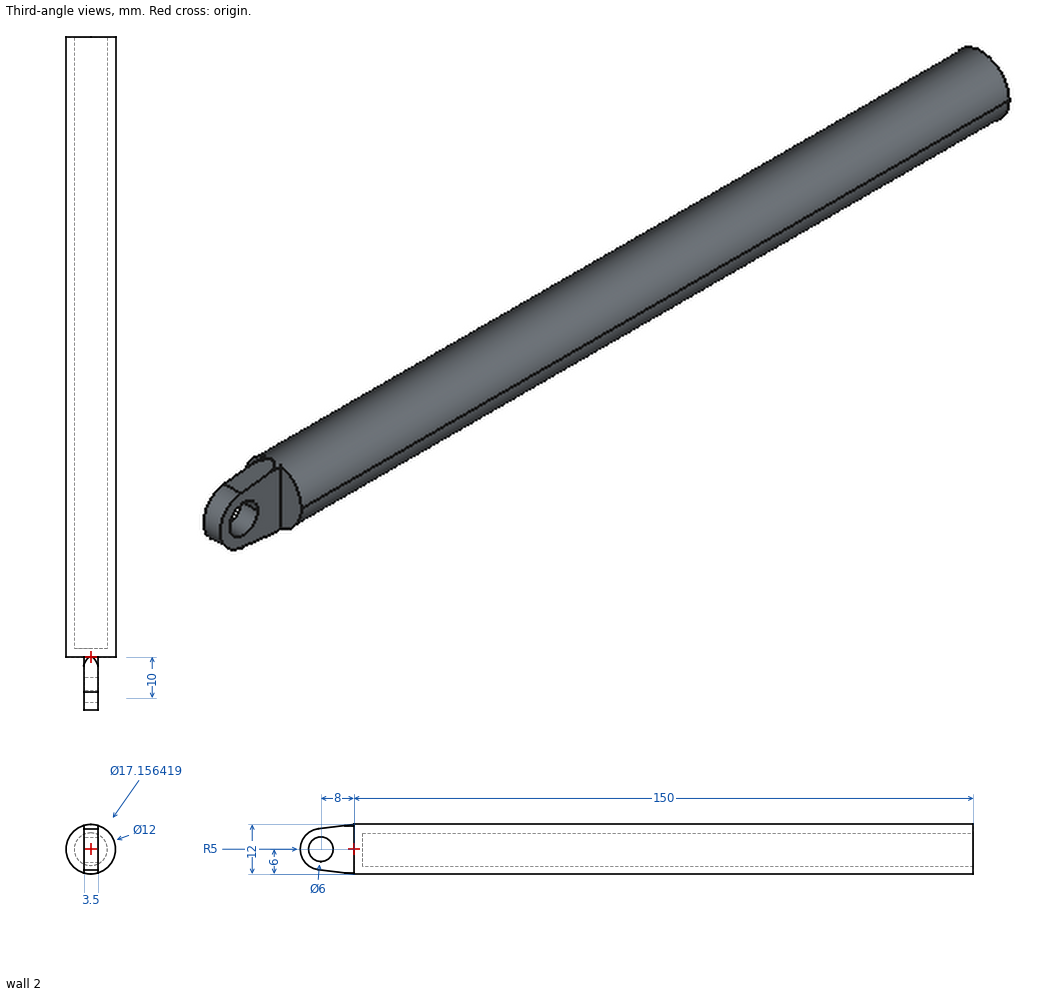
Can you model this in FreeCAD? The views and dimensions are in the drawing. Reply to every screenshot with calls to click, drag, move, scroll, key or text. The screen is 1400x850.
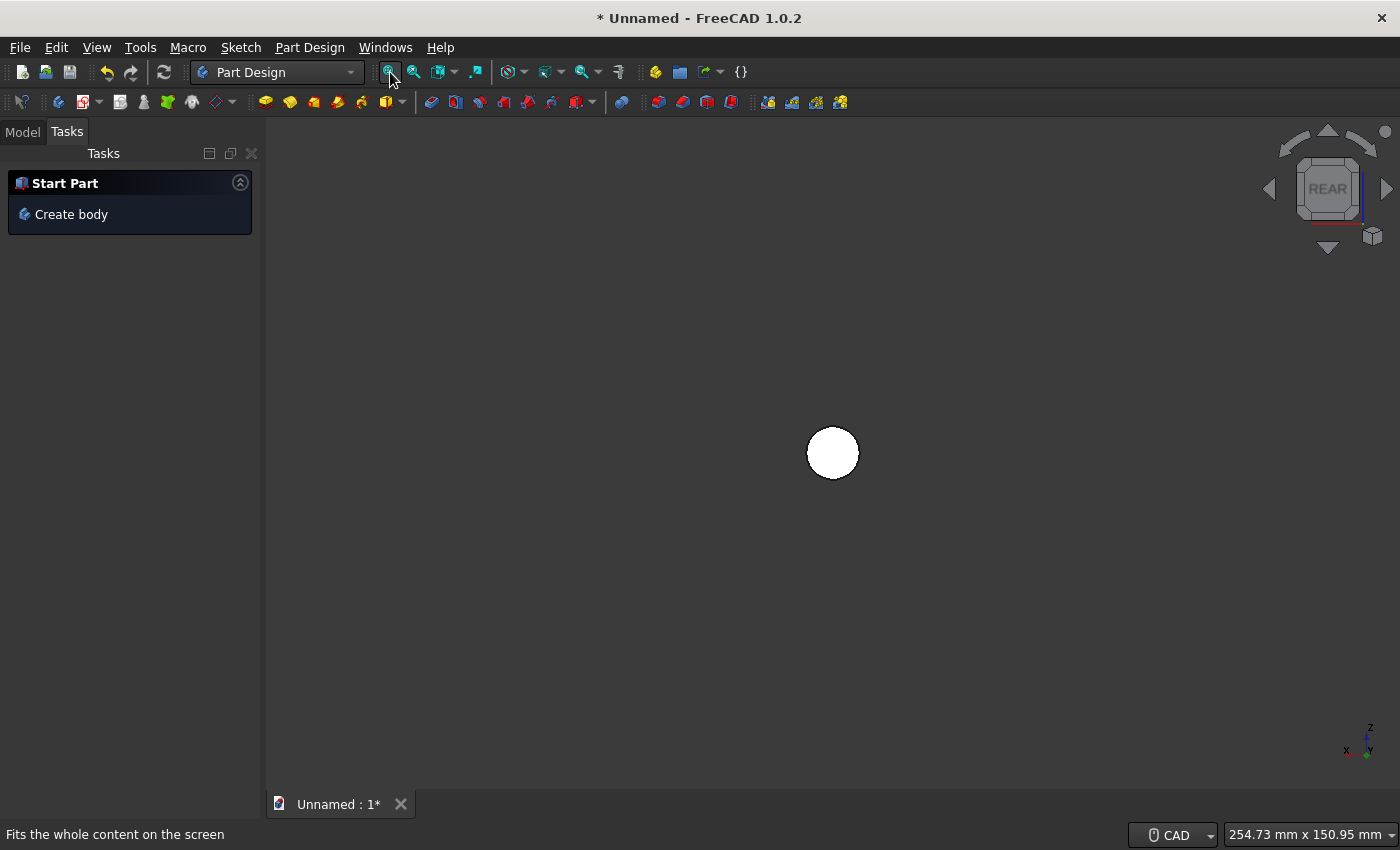
click(833, 452)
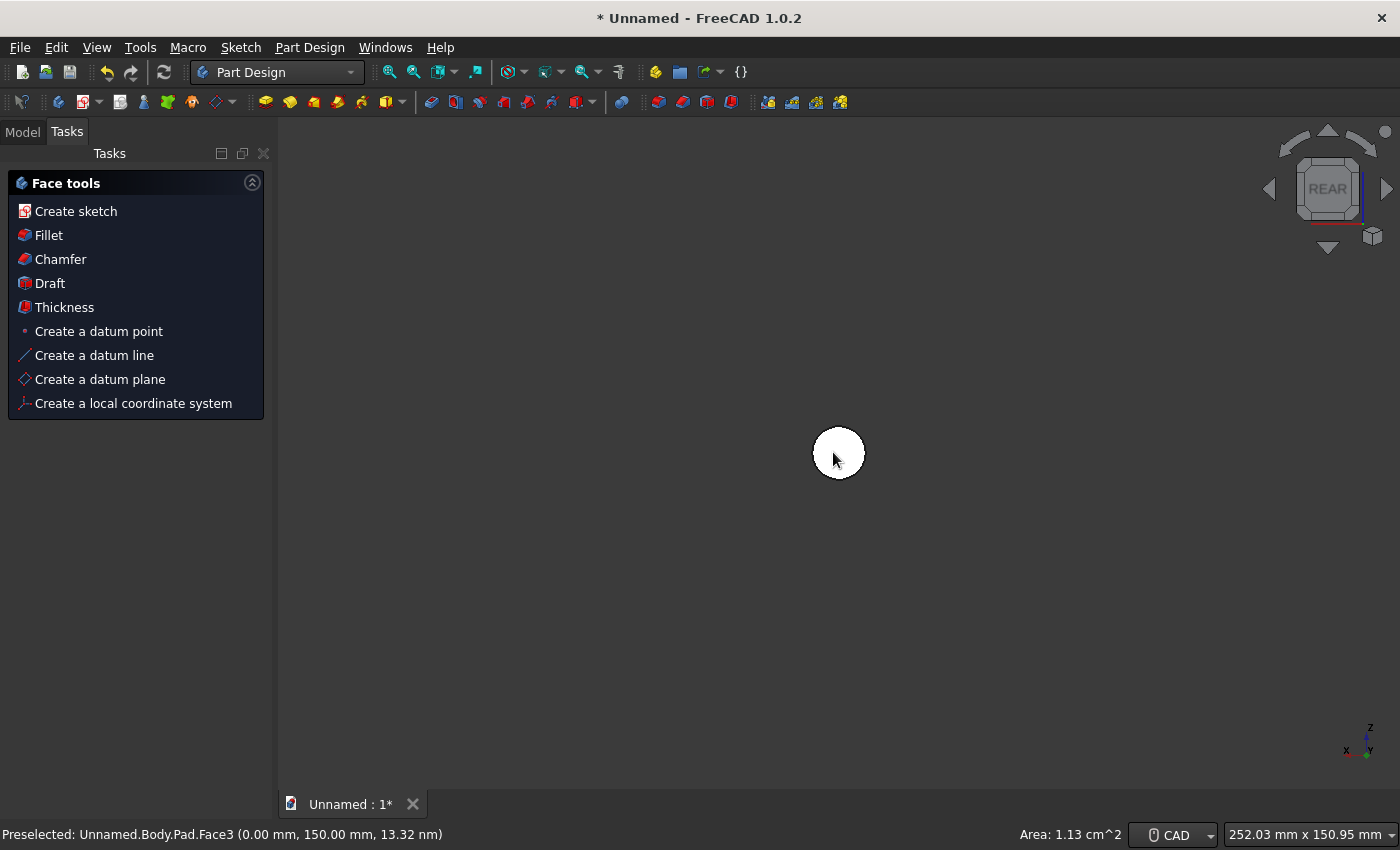
click(732, 102)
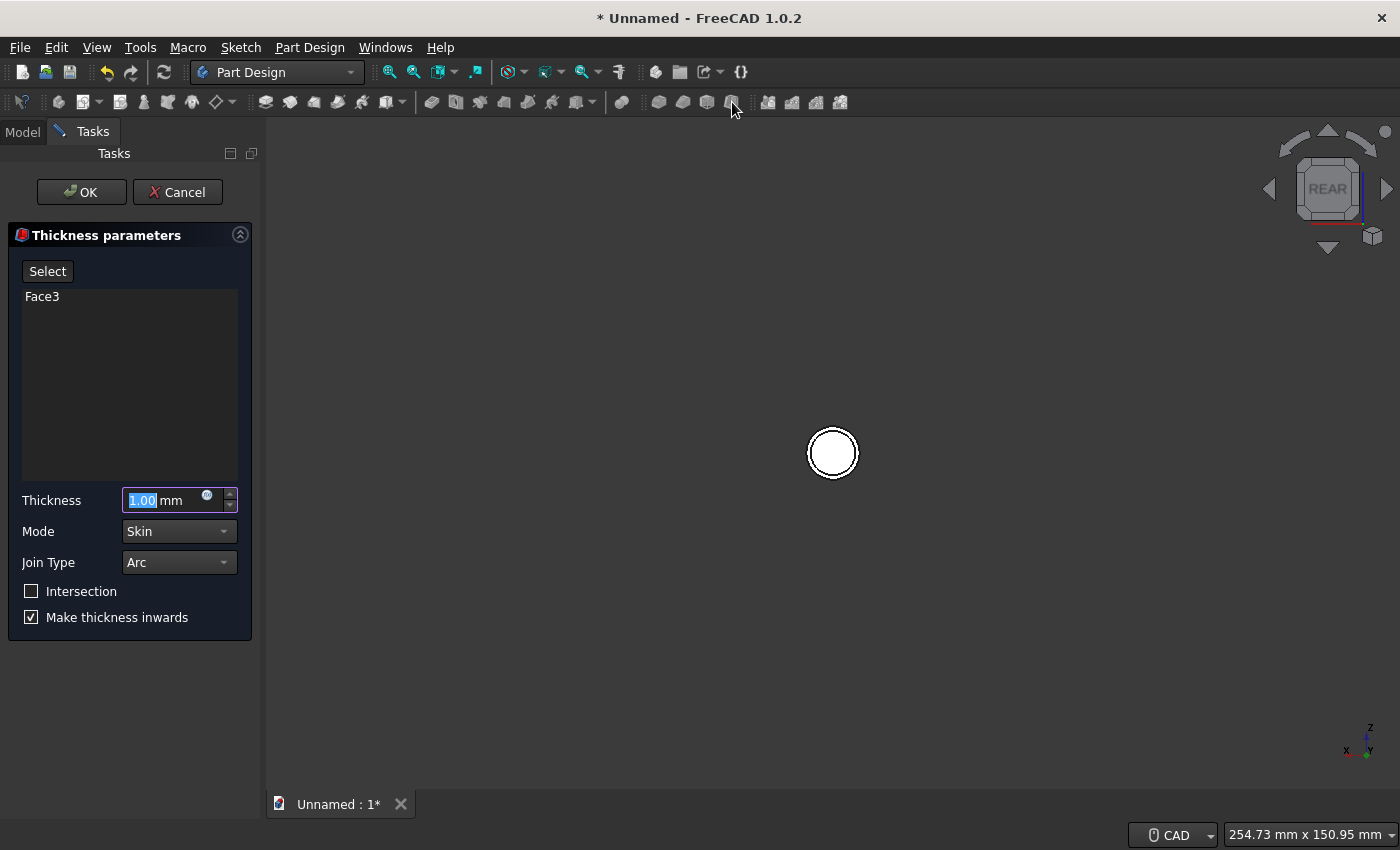
text(2)
key(Tab)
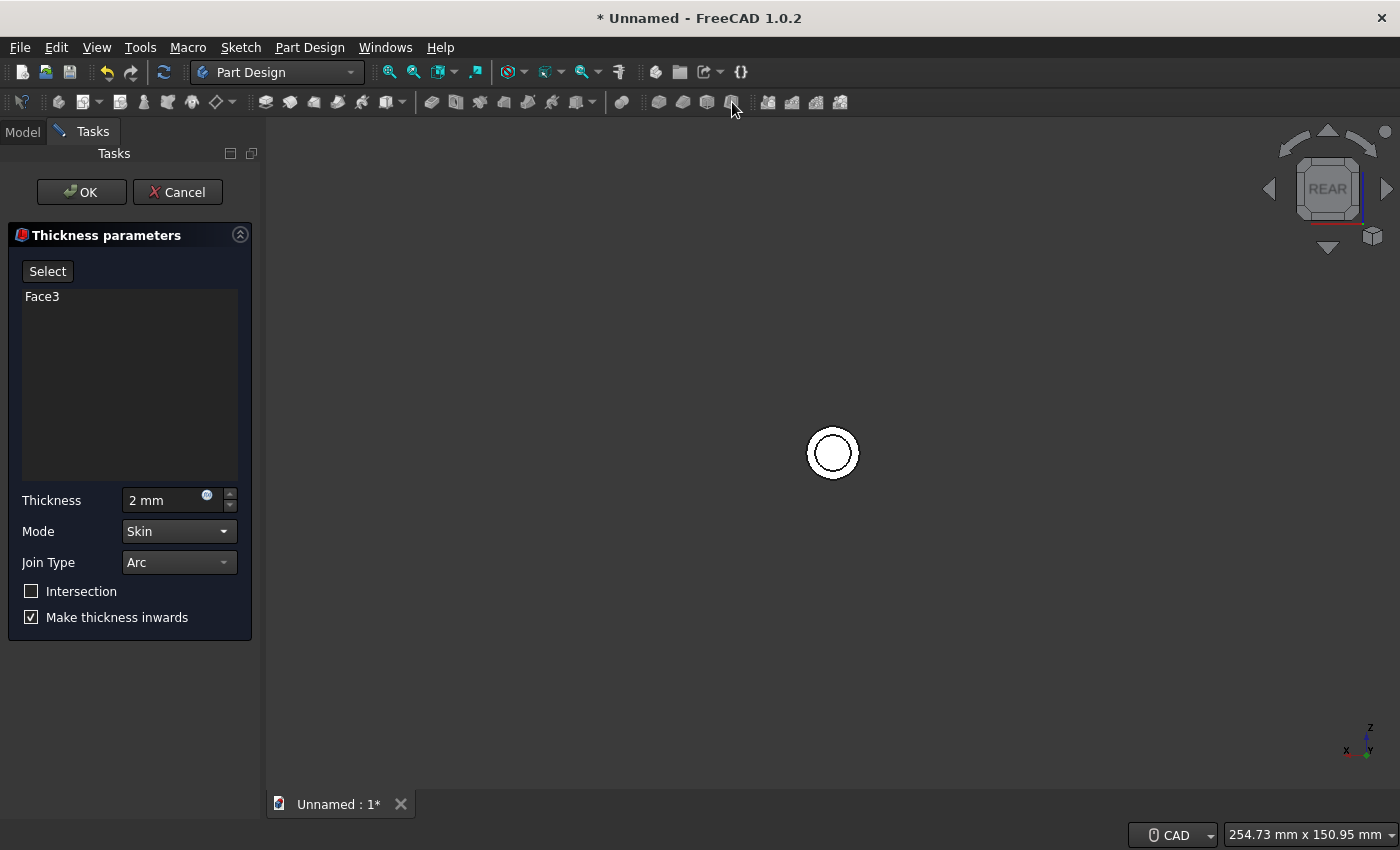
click(180, 562)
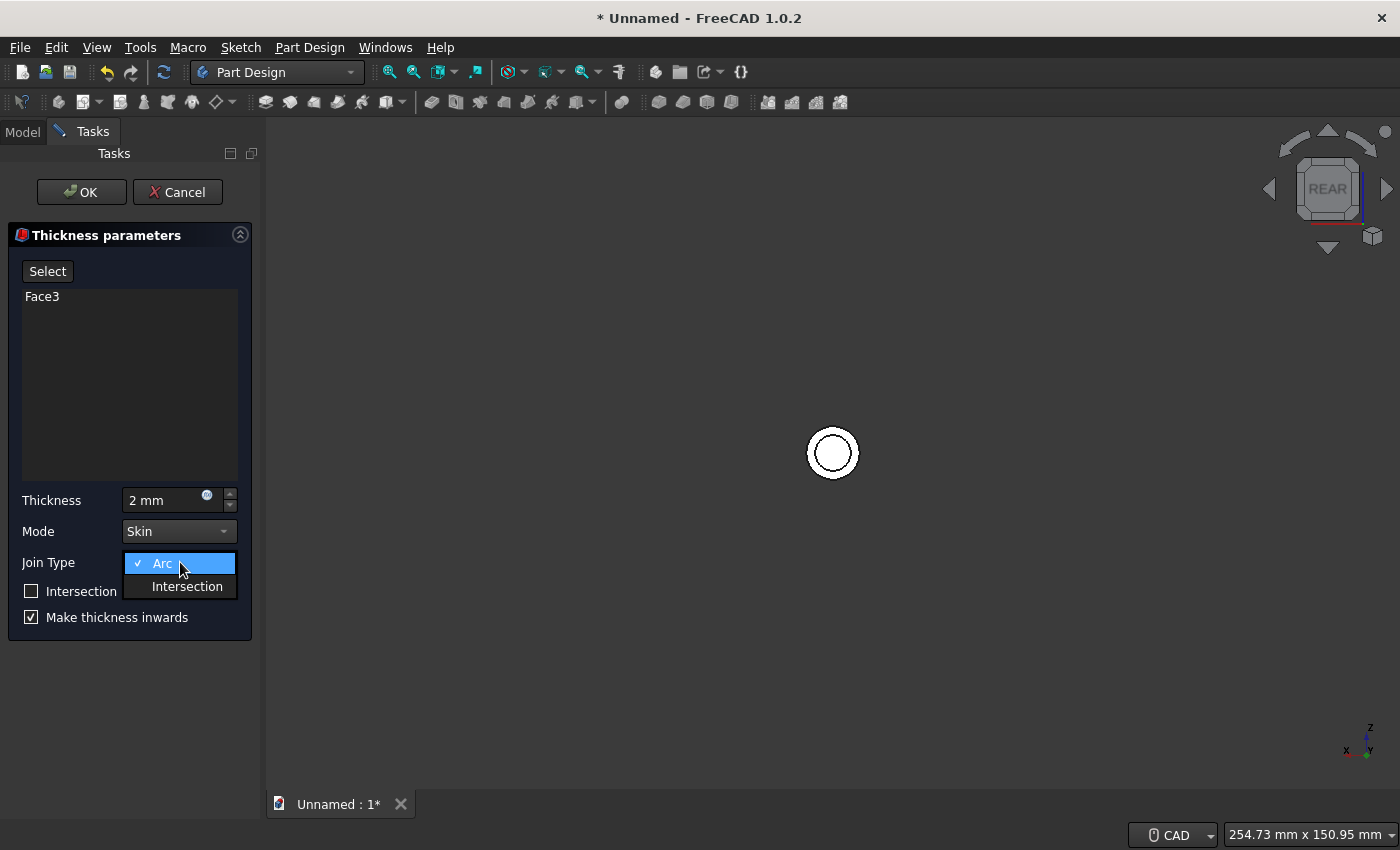
click(179, 586)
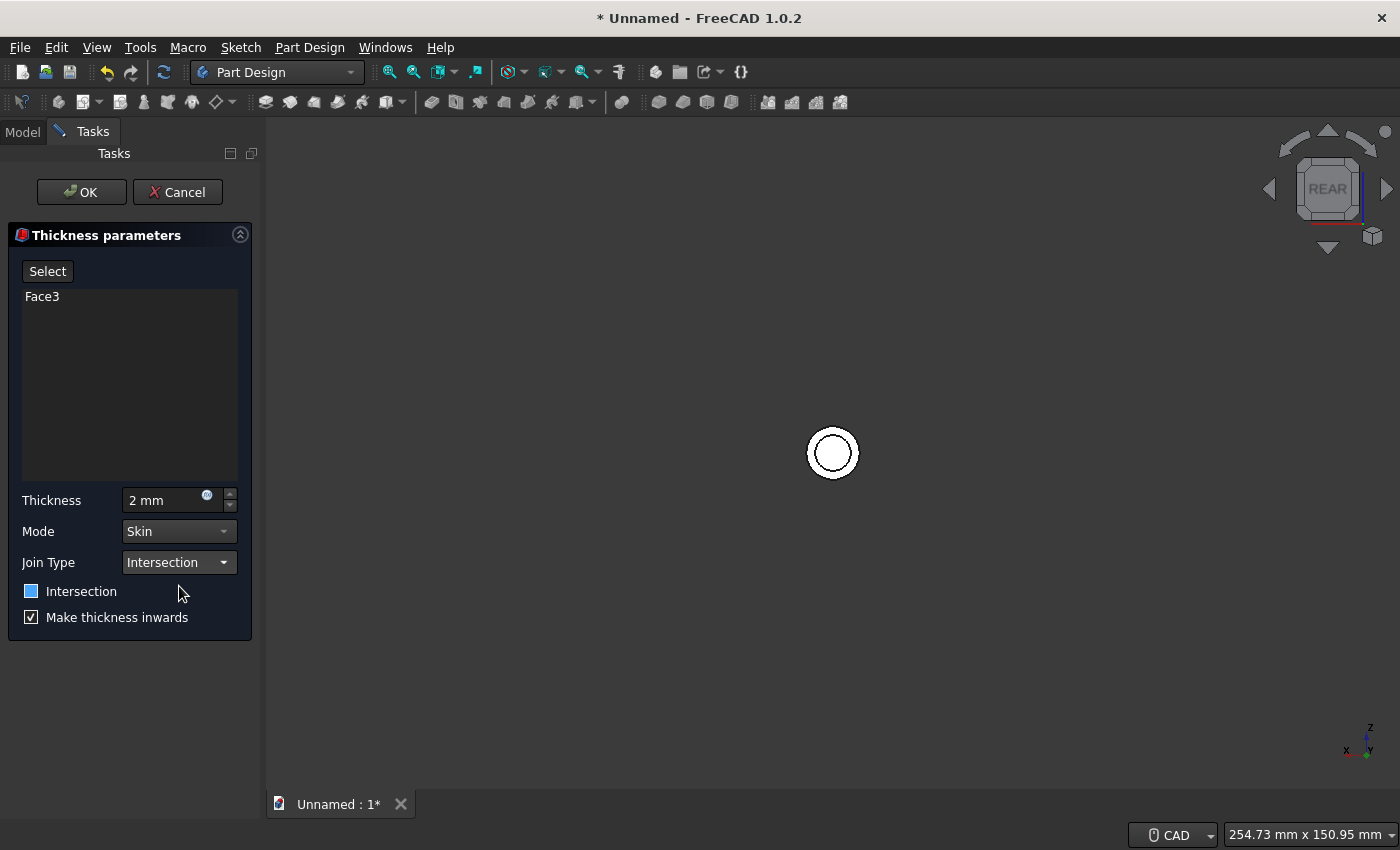
click(82, 192)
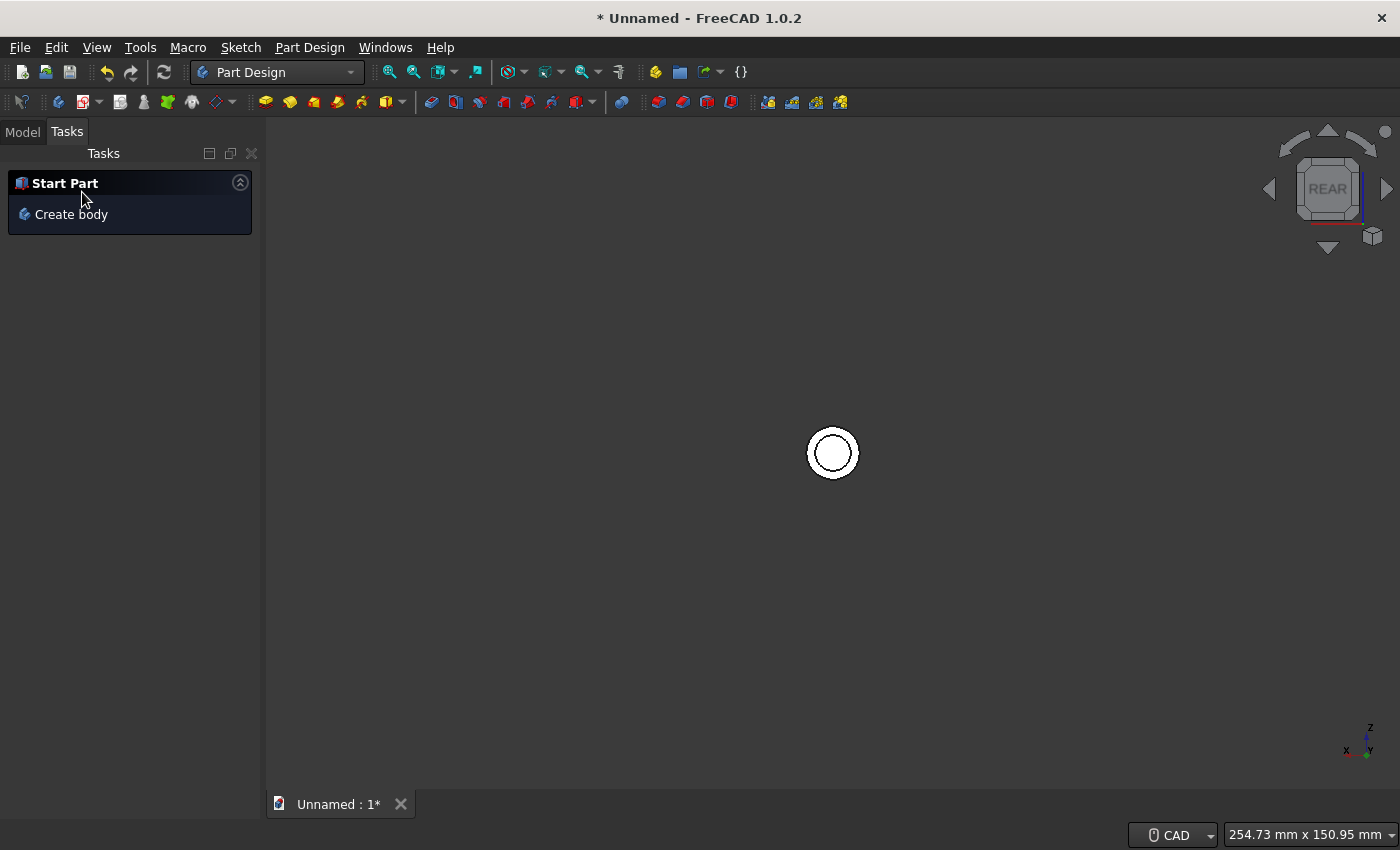
click(390, 72)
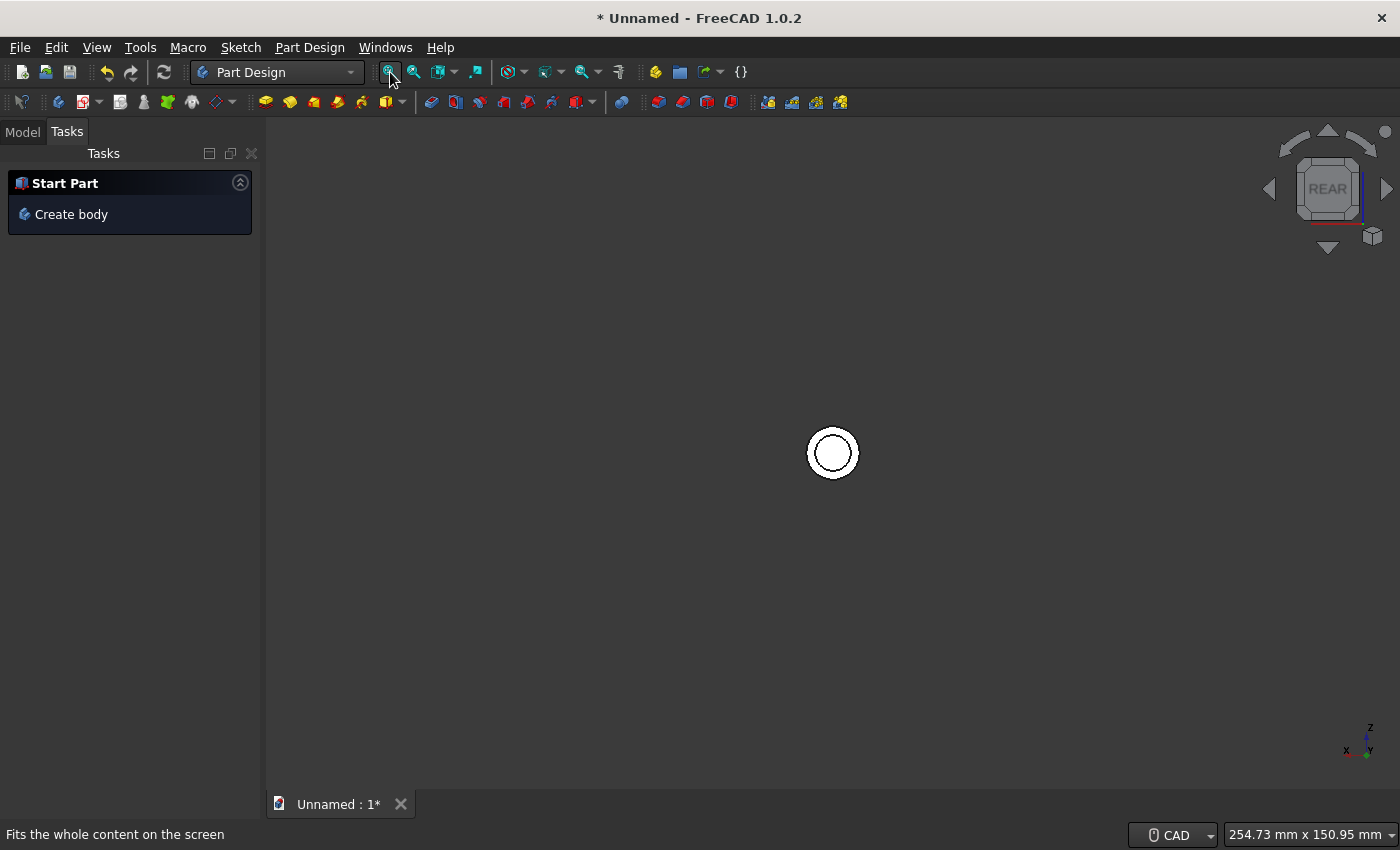
click(84, 102)